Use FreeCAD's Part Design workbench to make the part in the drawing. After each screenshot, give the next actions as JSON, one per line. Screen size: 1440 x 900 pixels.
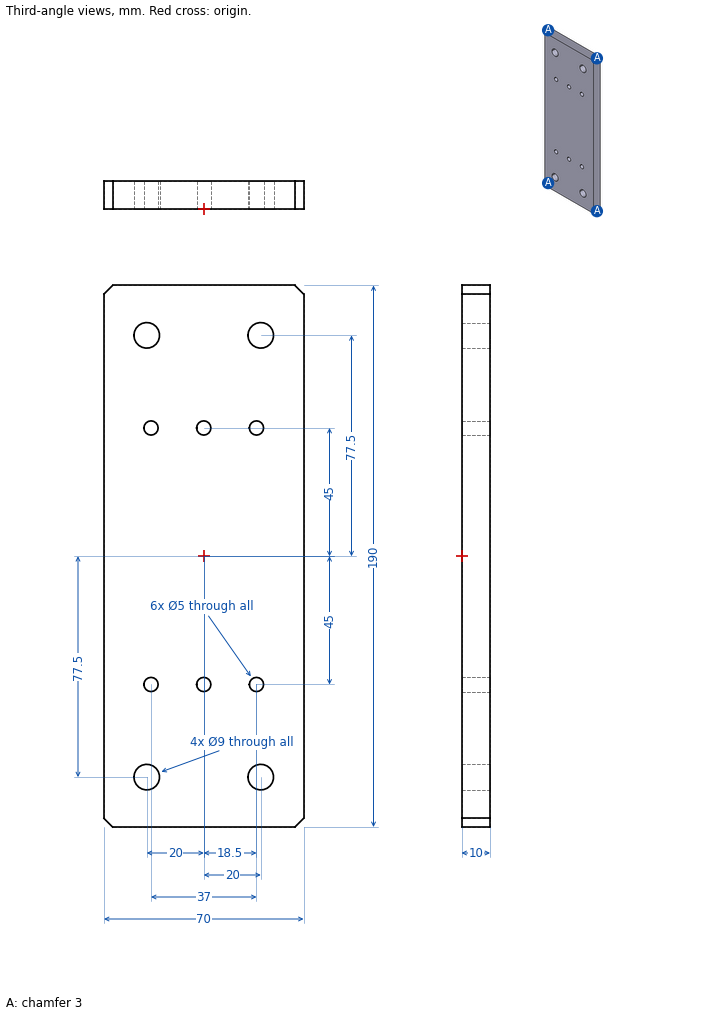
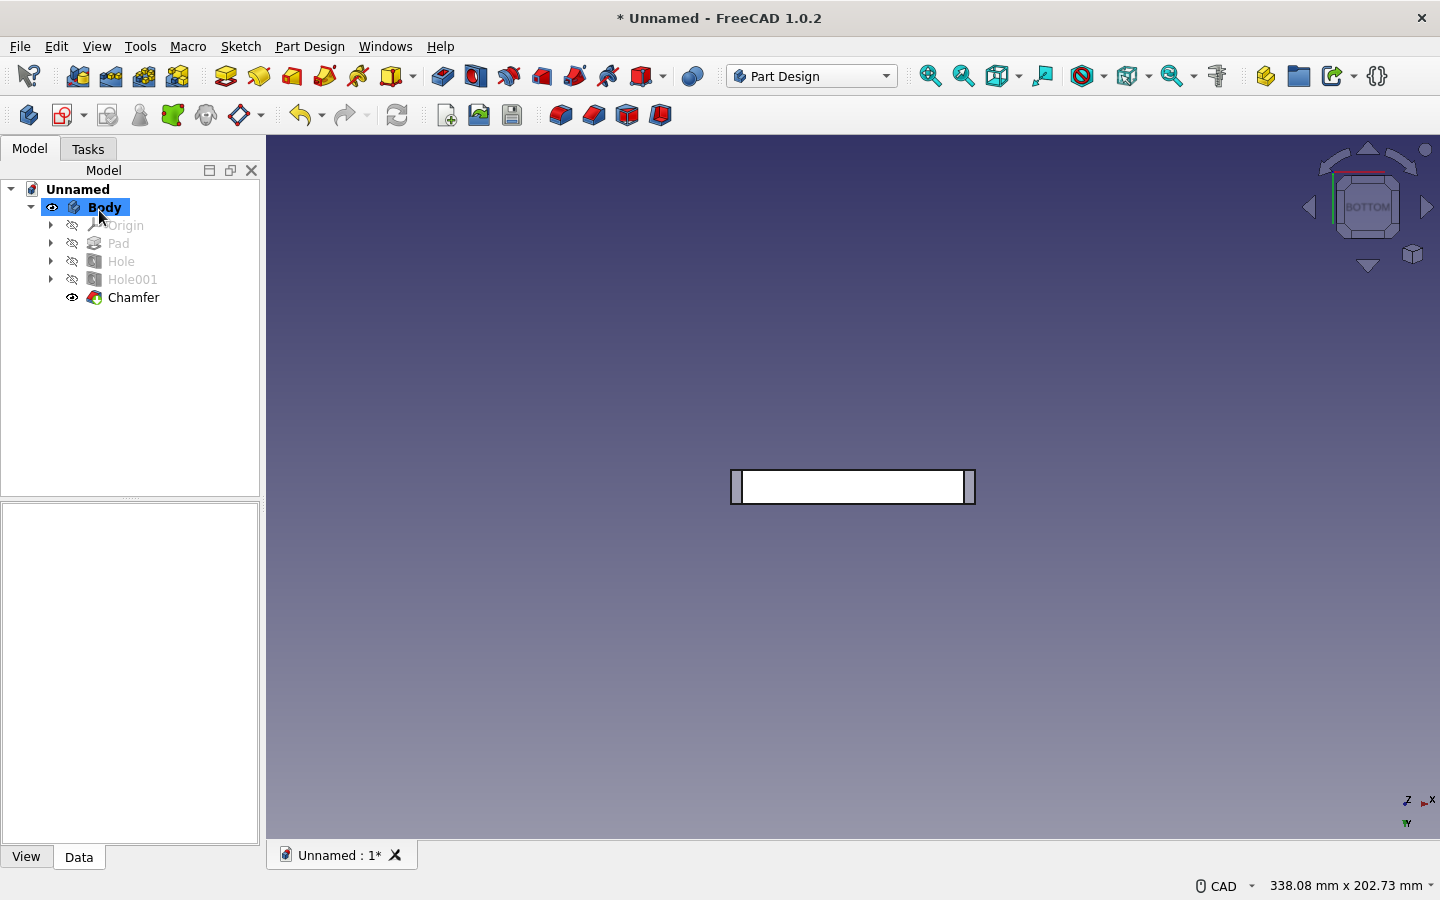
{"action": "key", "text": "0"}